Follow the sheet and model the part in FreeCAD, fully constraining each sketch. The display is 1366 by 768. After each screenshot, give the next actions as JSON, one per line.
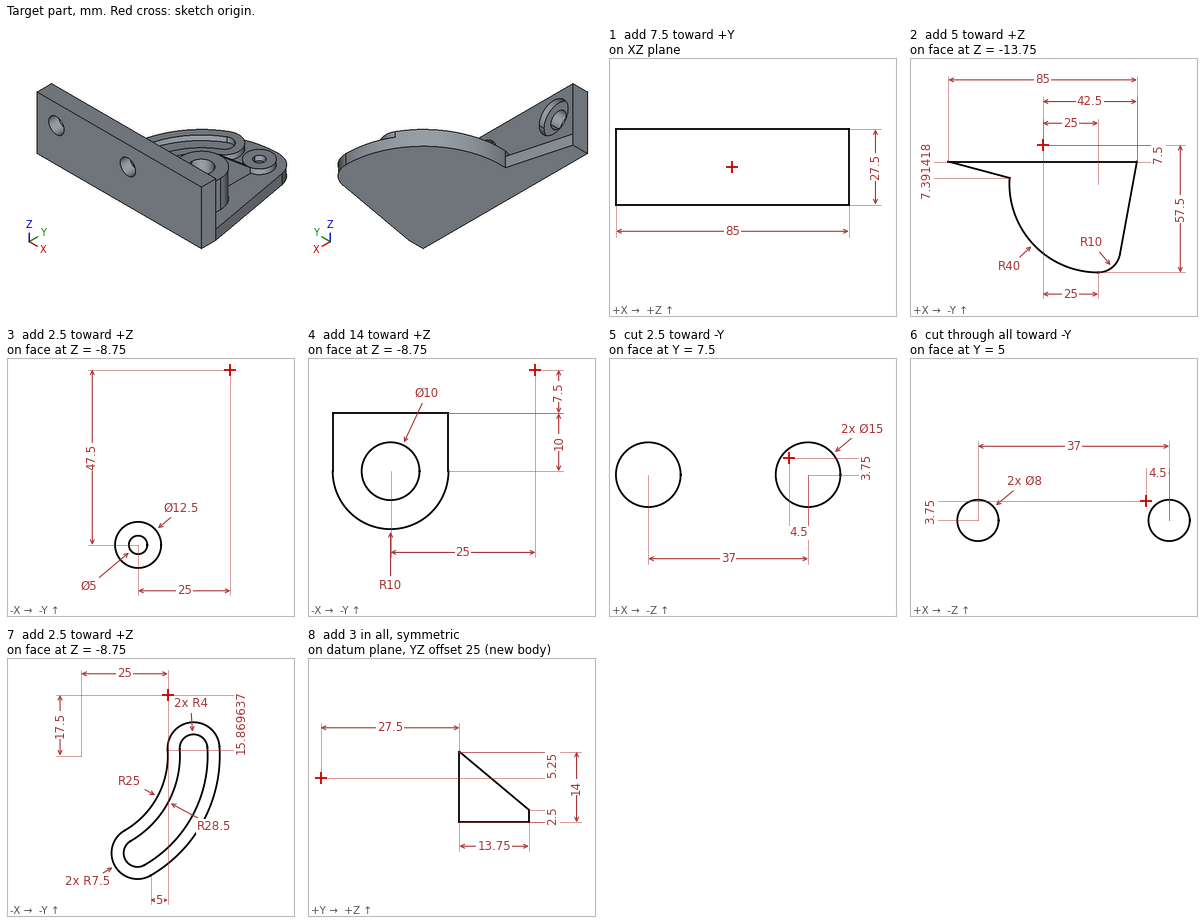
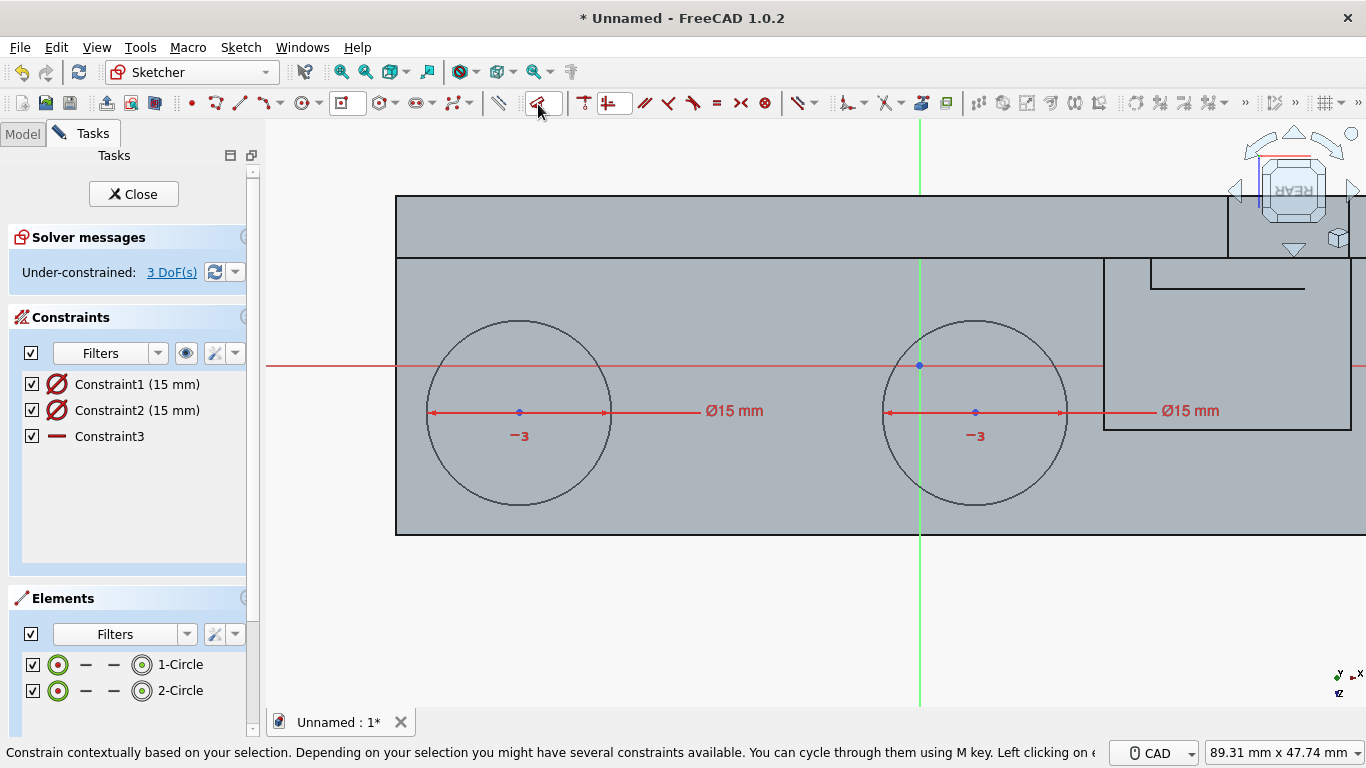
{"action": "left_click", "coordinate": [975, 413]}
{"action": "left_click", "coordinate": [947, 447]}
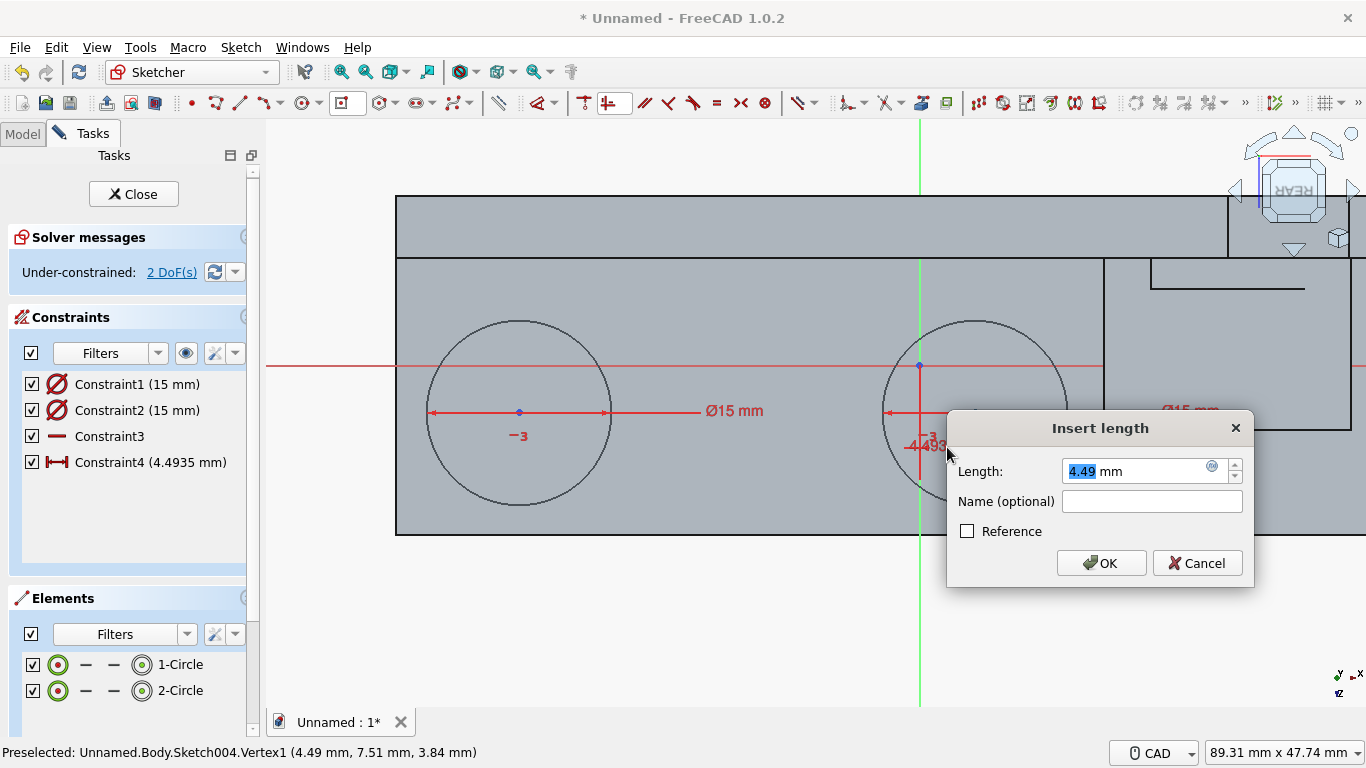
{"action": "type", "text": "4.5"}
{"action": "key", "text": "Return"}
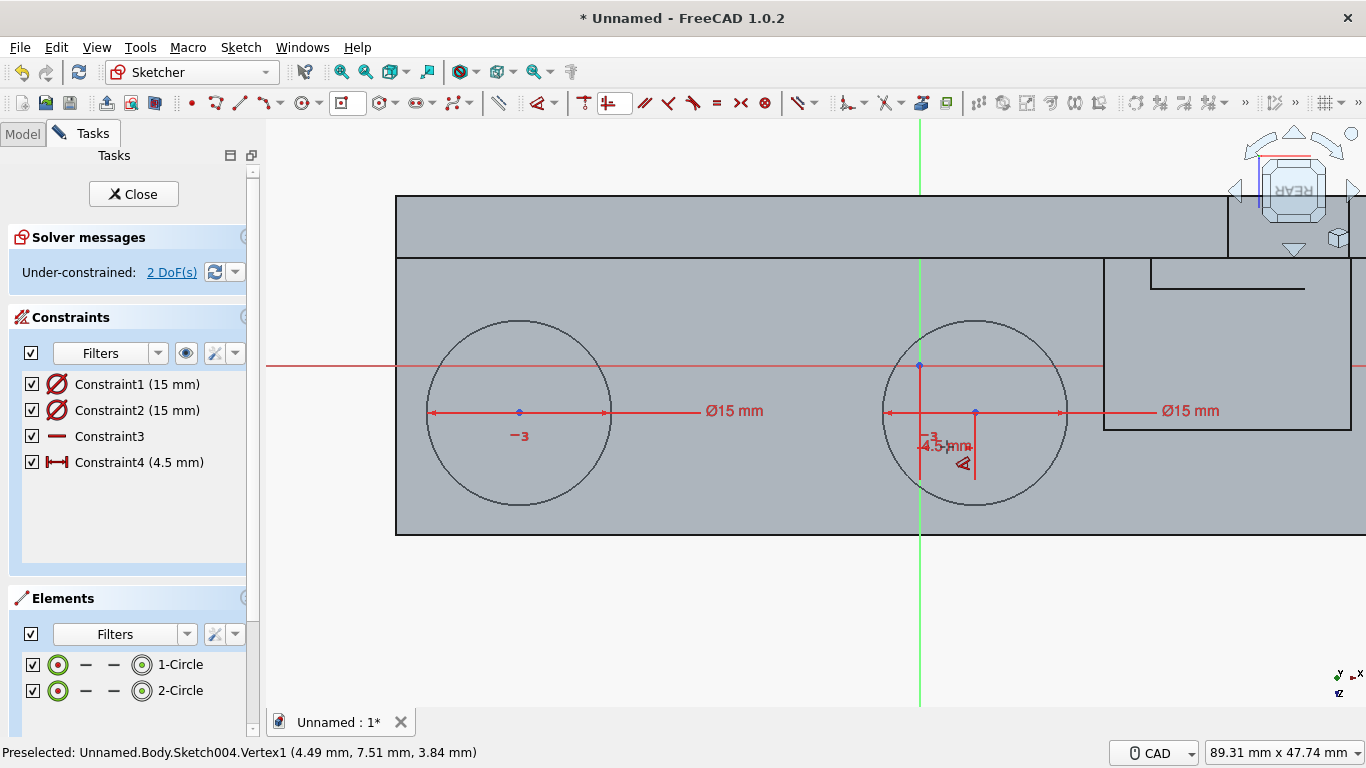
{"action": "left_click", "coordinate": [975, 413]}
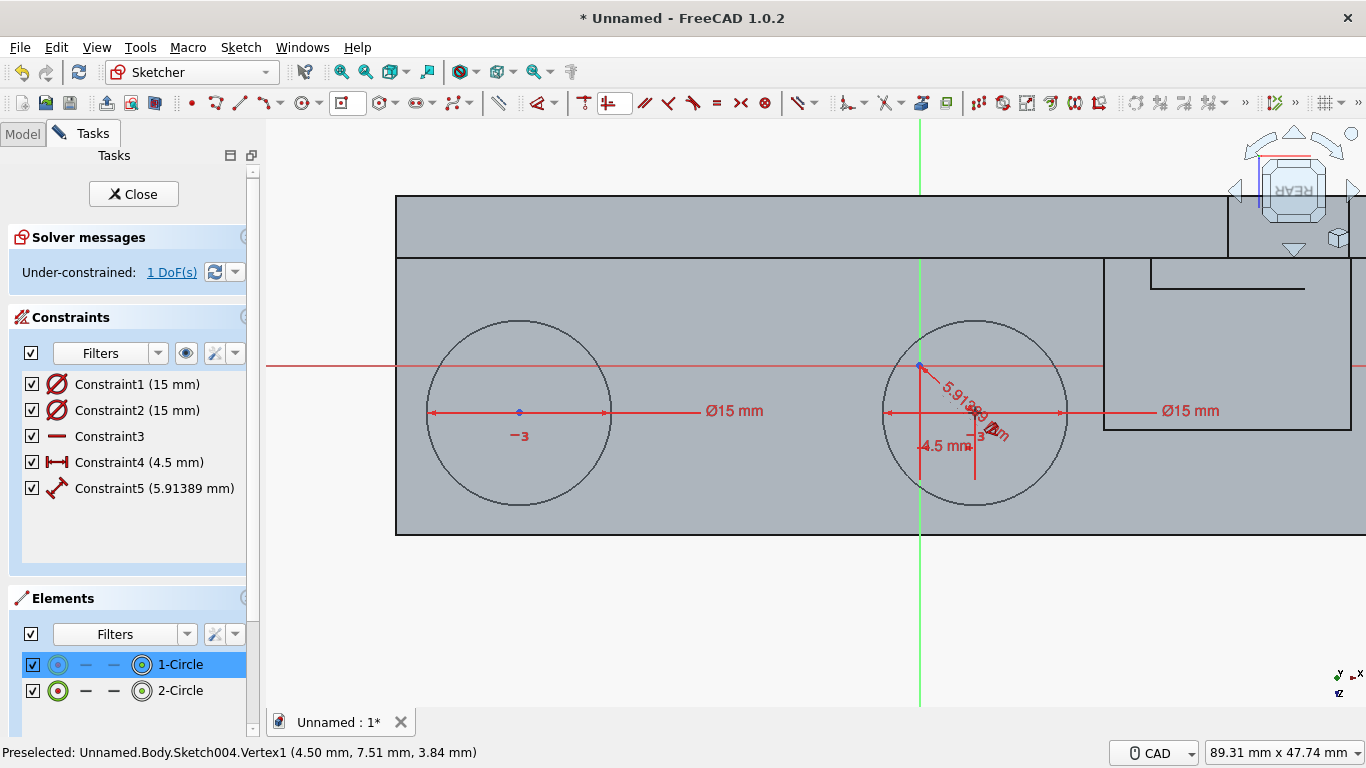
{"action": "left_click", "coordinate": [519, 413]}
{"action": "left_click", "coordinate": [747, 447]}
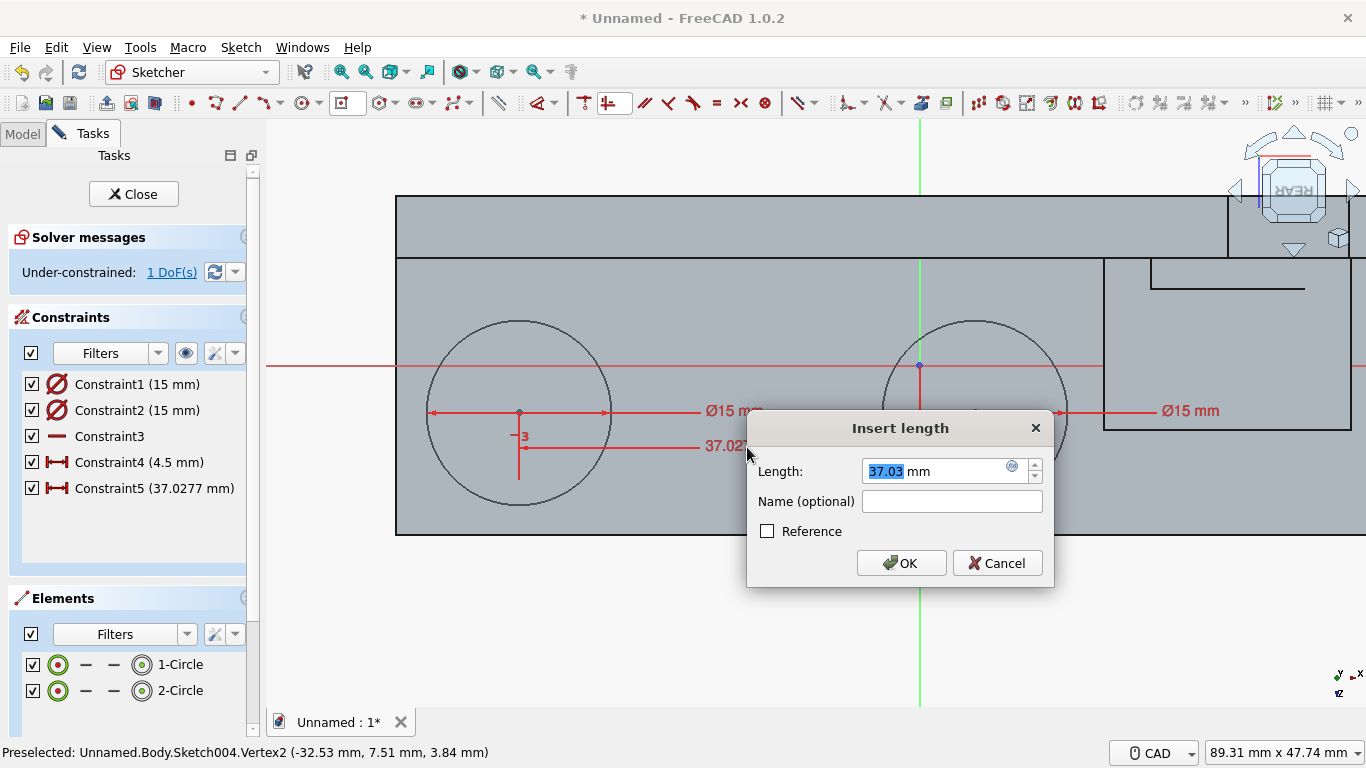
{"action": "type", "text": "37"}
{"action": "key", "text": "Return"}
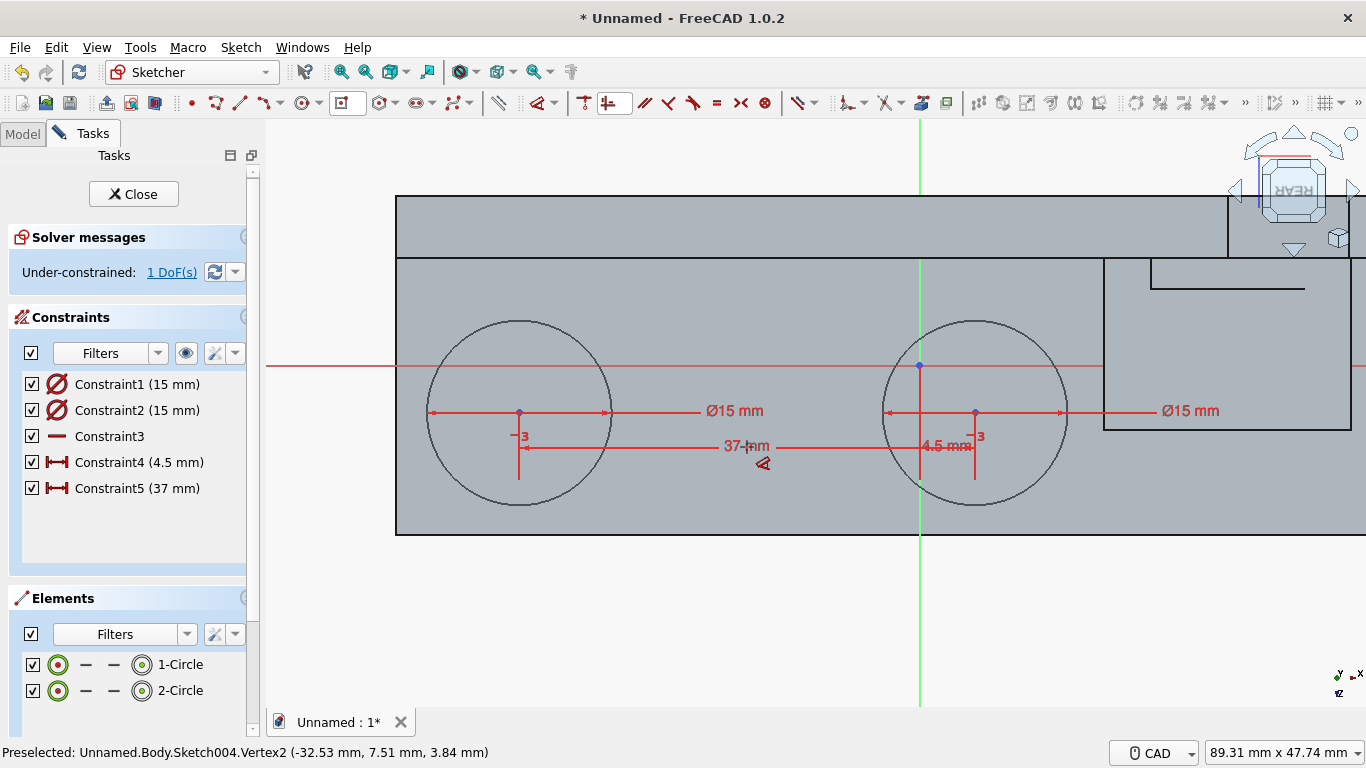
{"action": "left_click", "coordinate": [975, 413]}
{"action": "left_click", "coordinate": [1009, 389]}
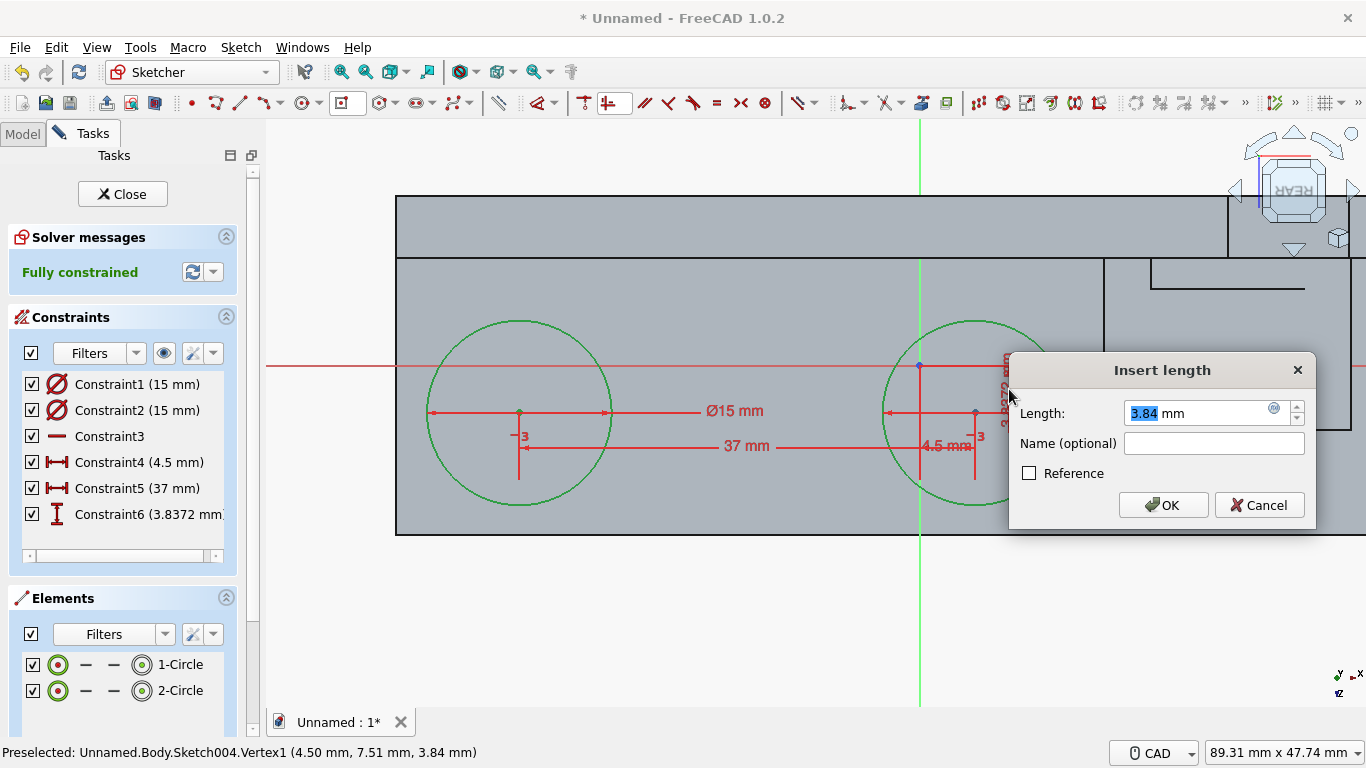
{"action": "type", "text": "3.75"}
{"action": "key", "text": "Return"}
{"action": "key", "text": "Escape"}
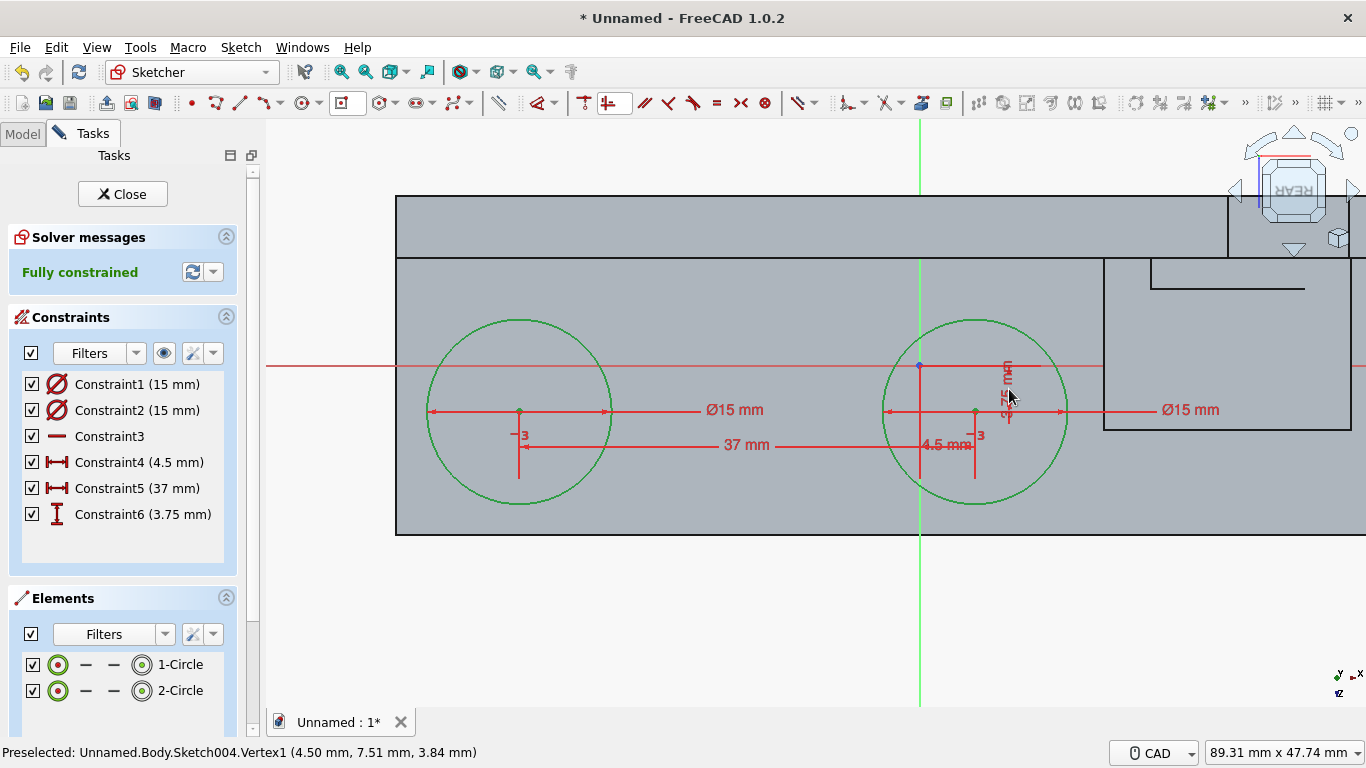
{"action": "left_click", "coordinate": [123, 194]}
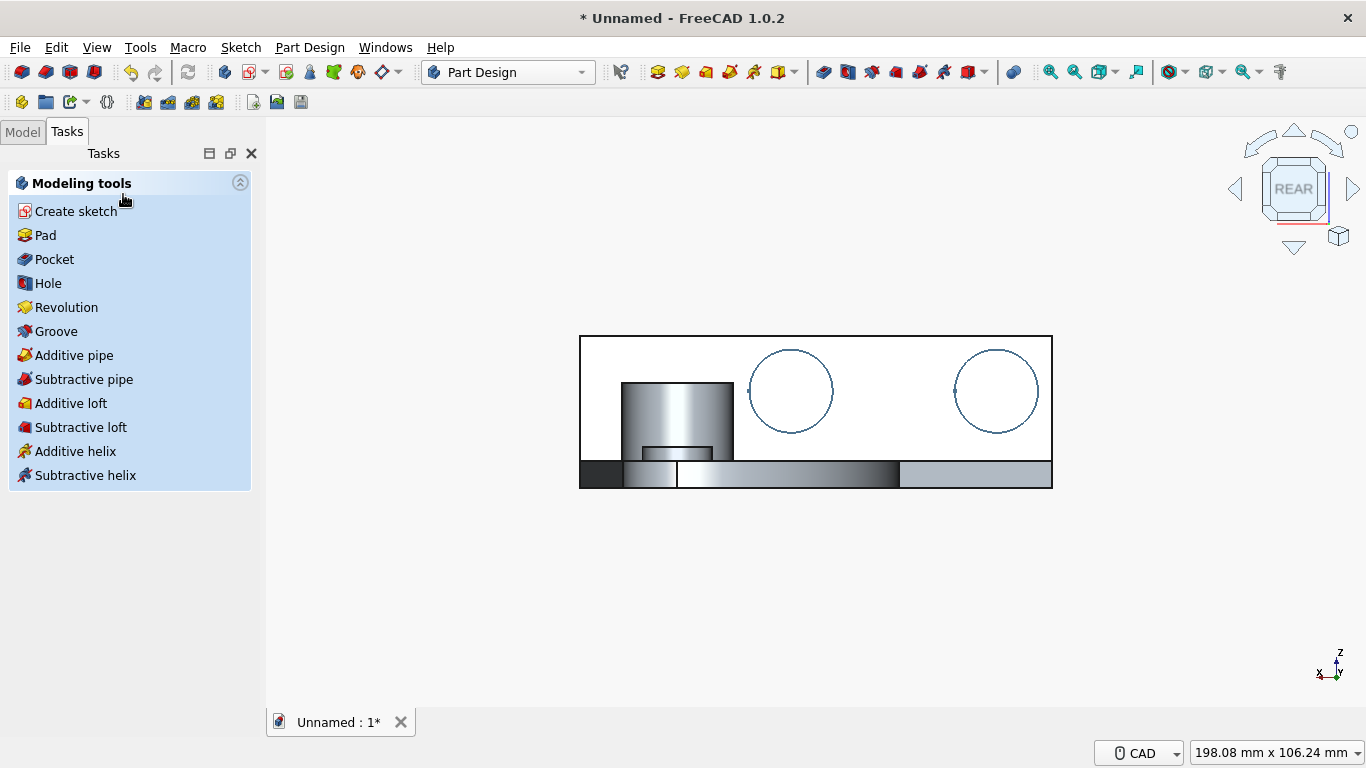
{"action": "left_click", "coordinate": [824, 72]}